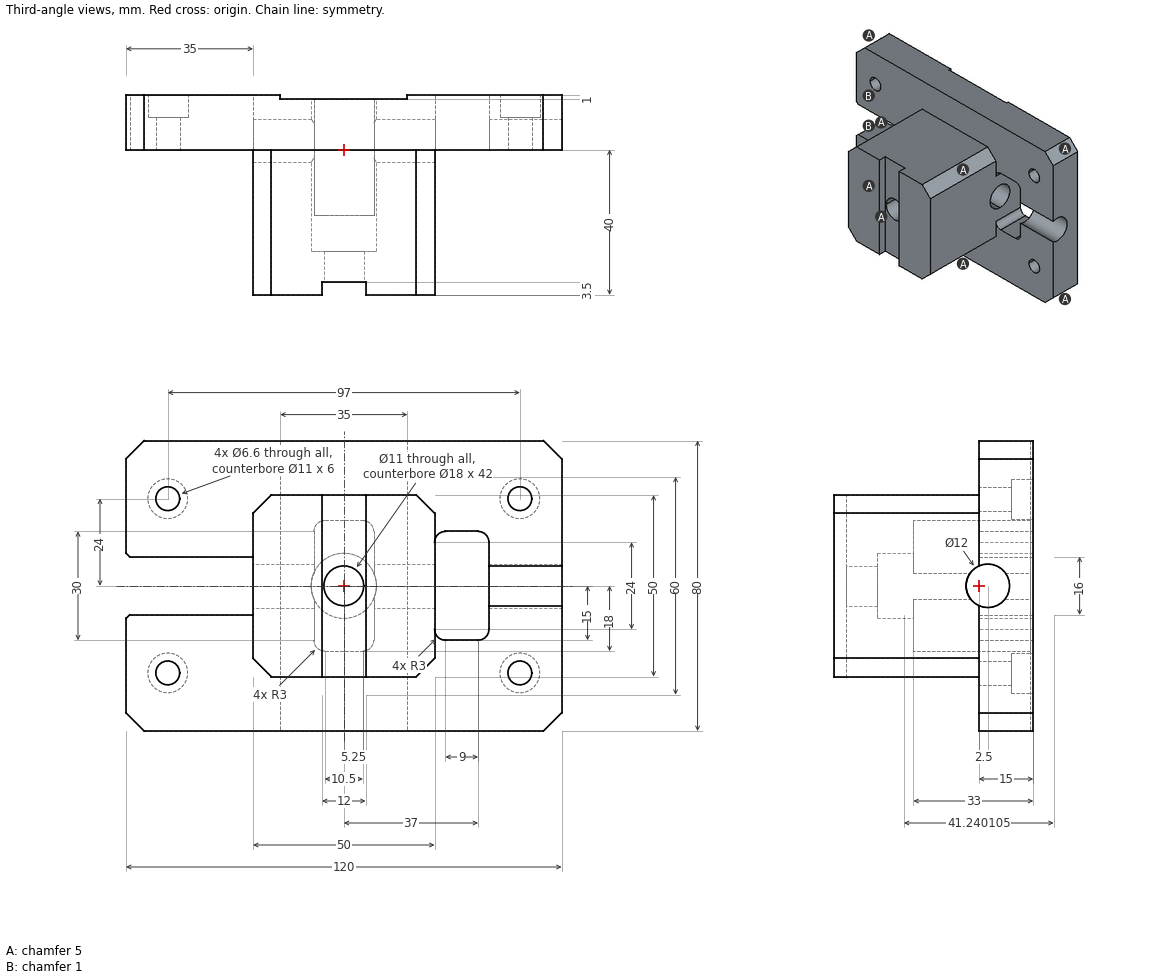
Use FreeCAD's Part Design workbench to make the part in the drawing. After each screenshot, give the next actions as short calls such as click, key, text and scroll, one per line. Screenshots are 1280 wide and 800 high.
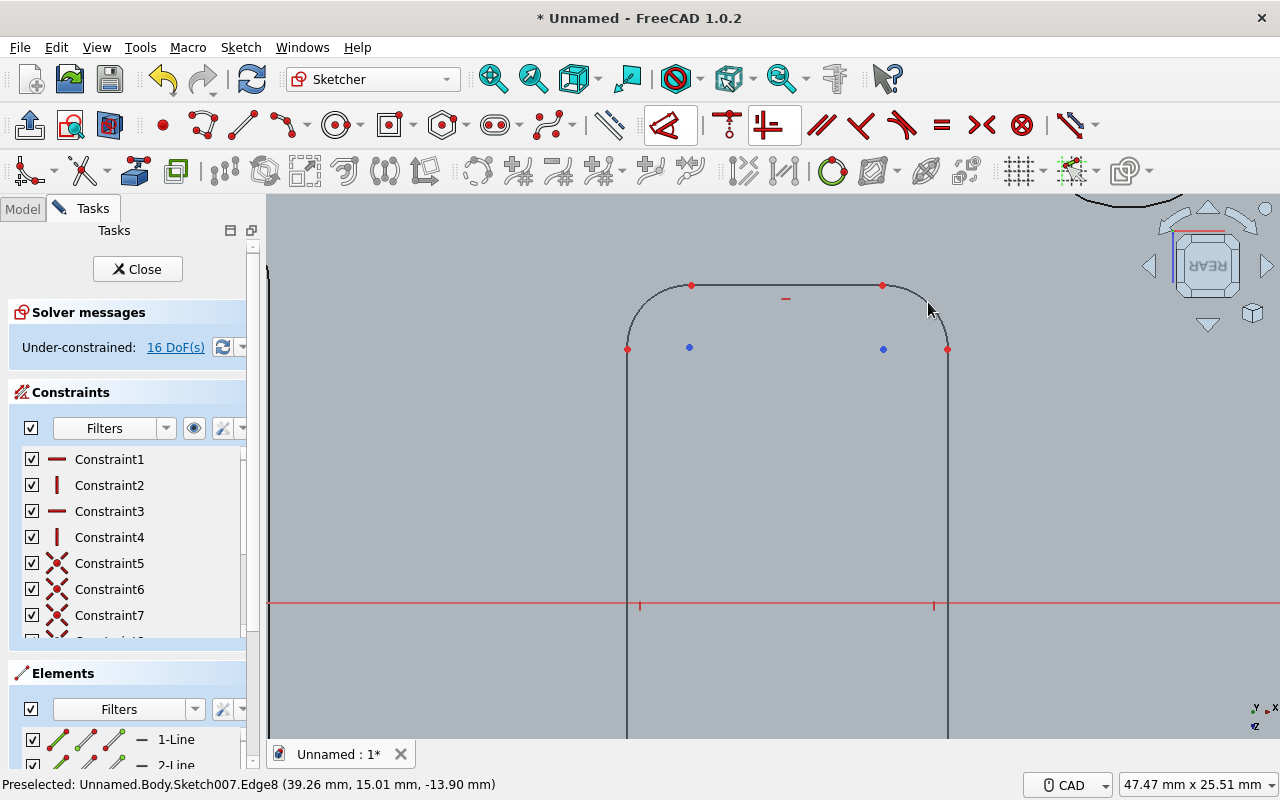
click(825, 285)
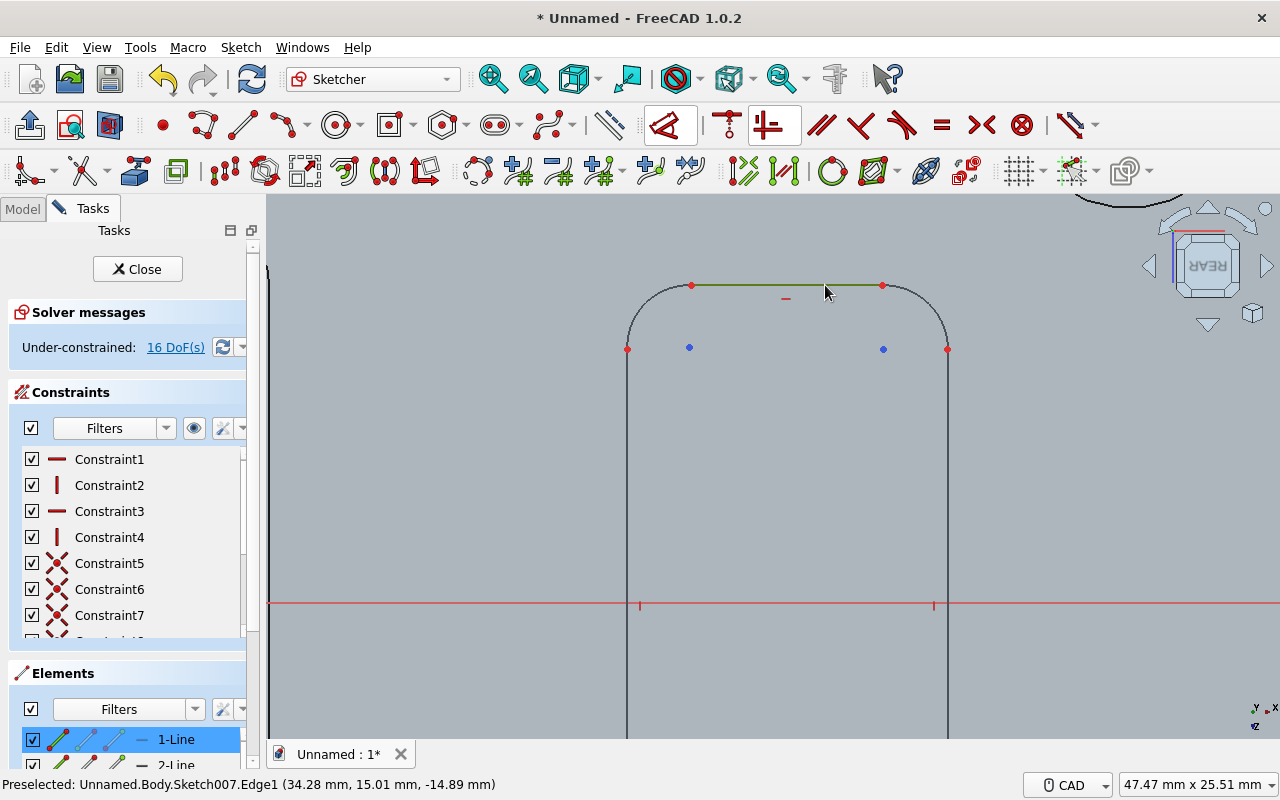
click(662, 292)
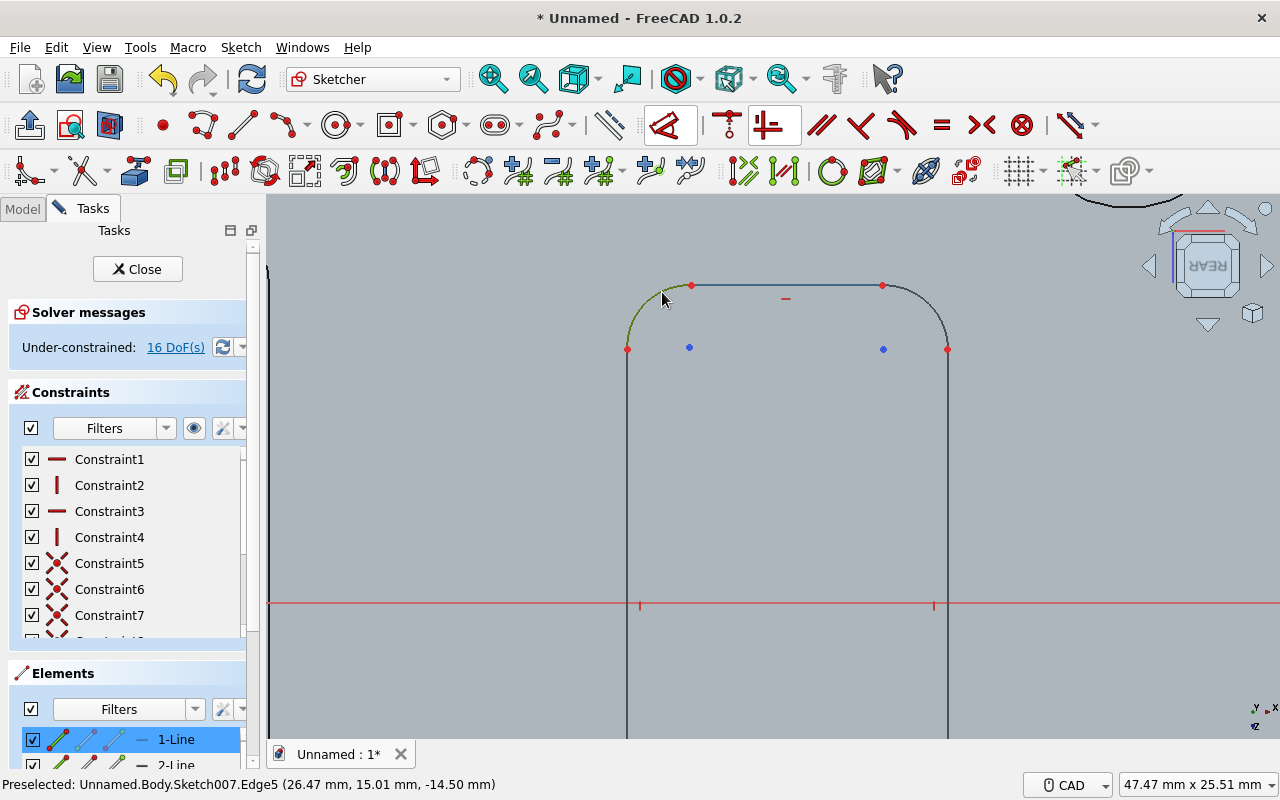
click(902, 126)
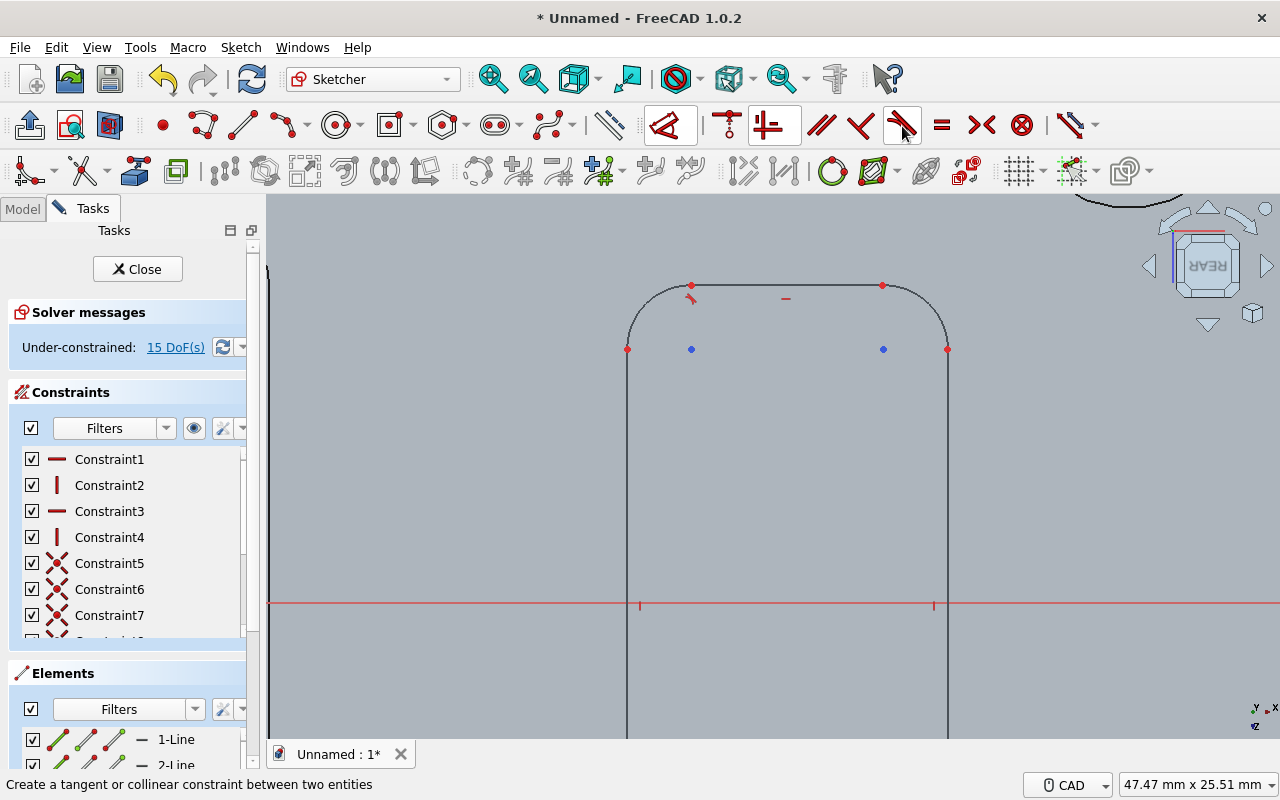
click(825, 285)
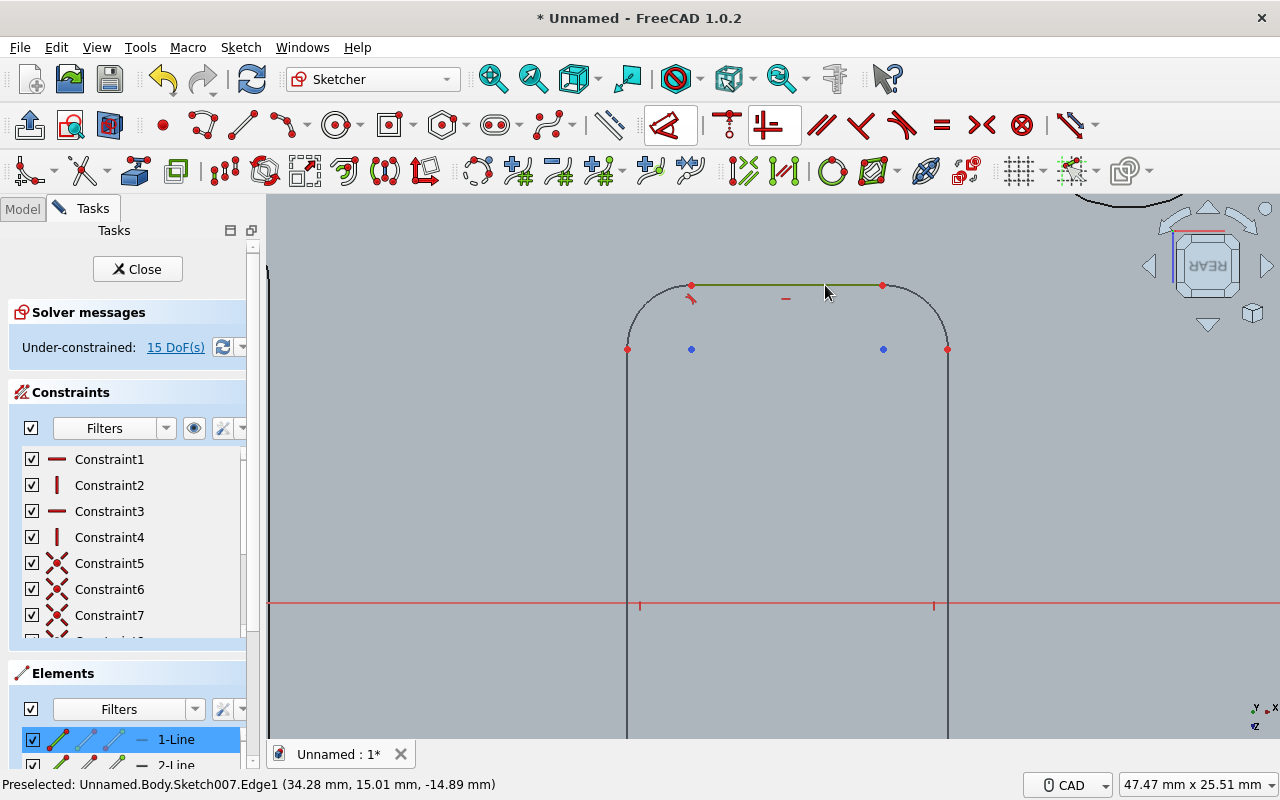
click(941, 320)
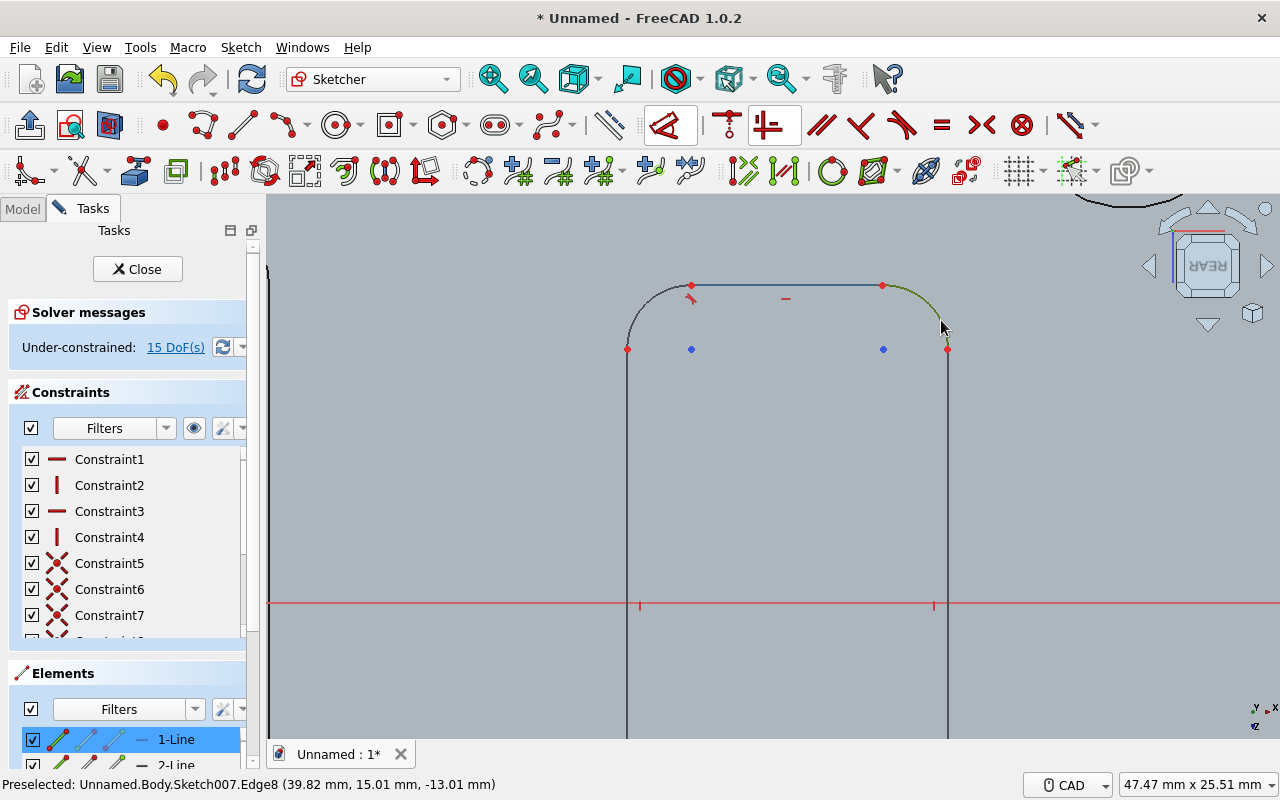
key(t)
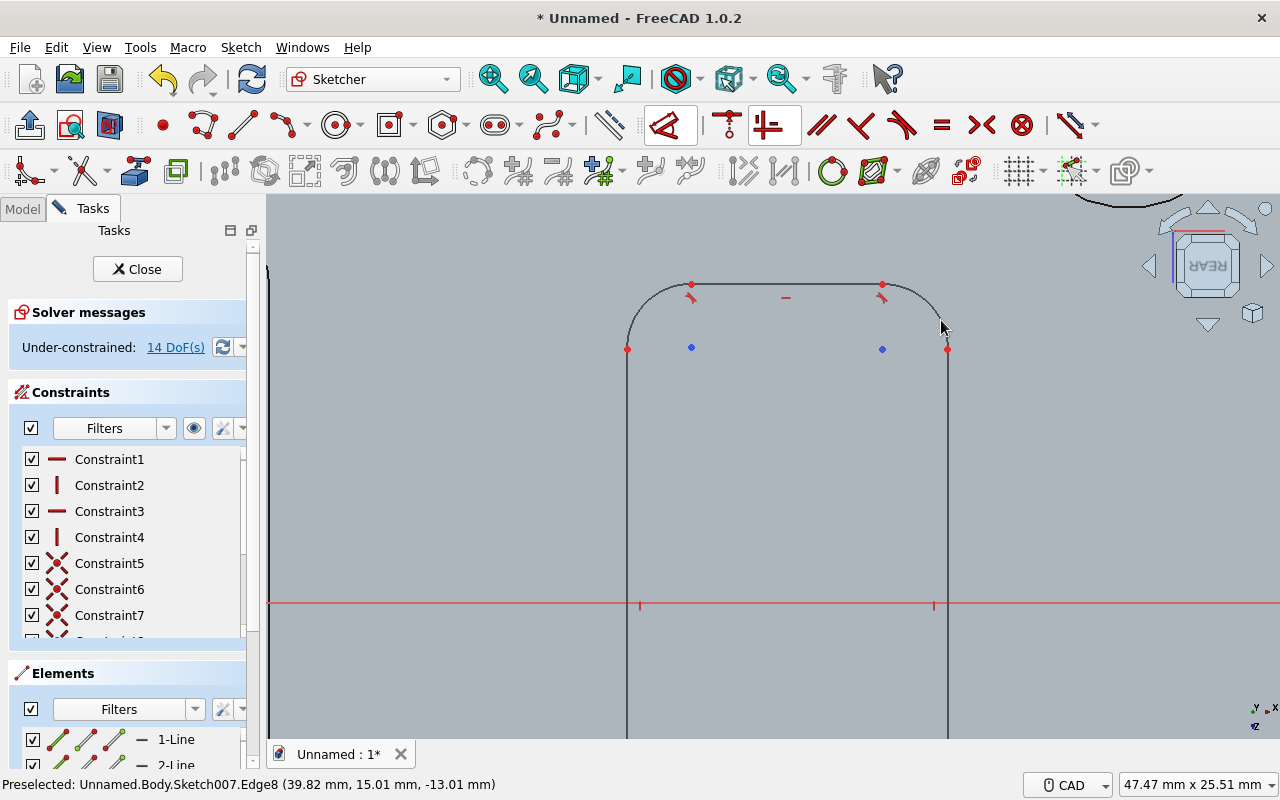
click(627, 503)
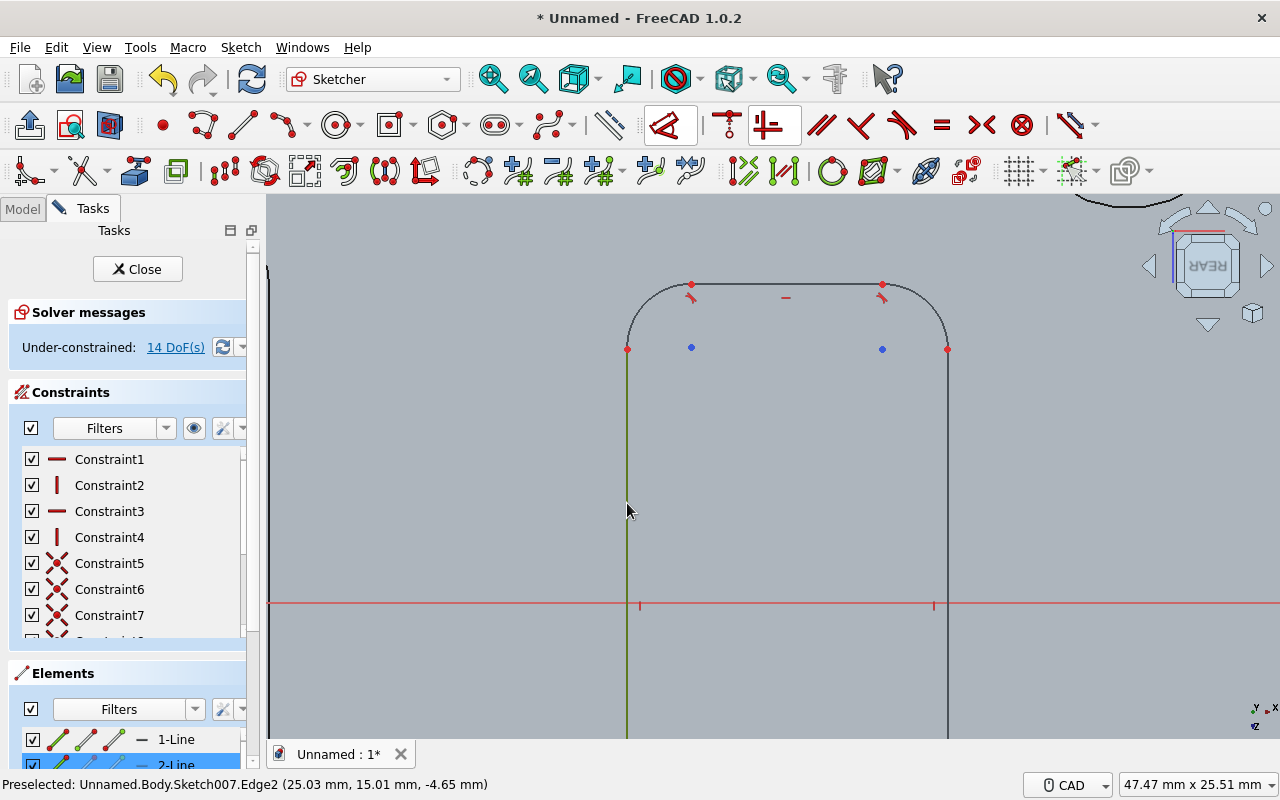
click(662, 291)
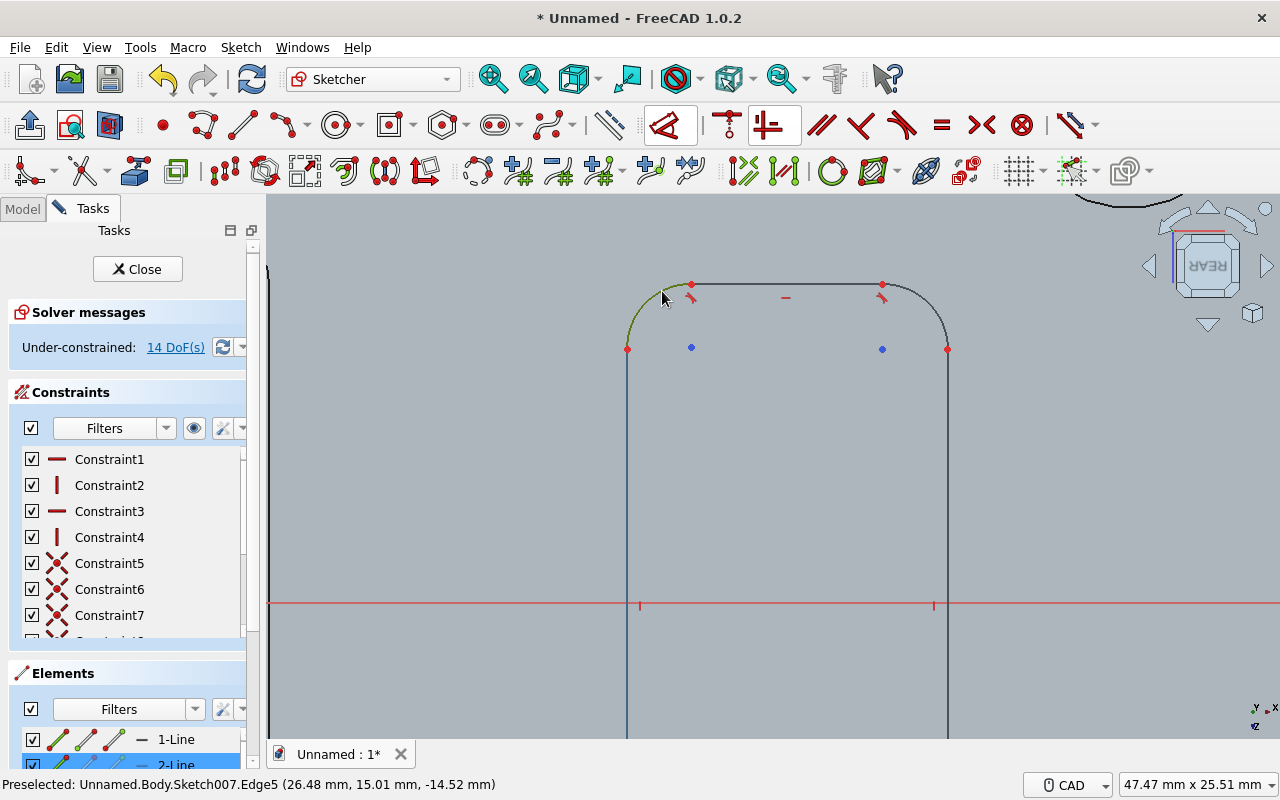
click(902, 126)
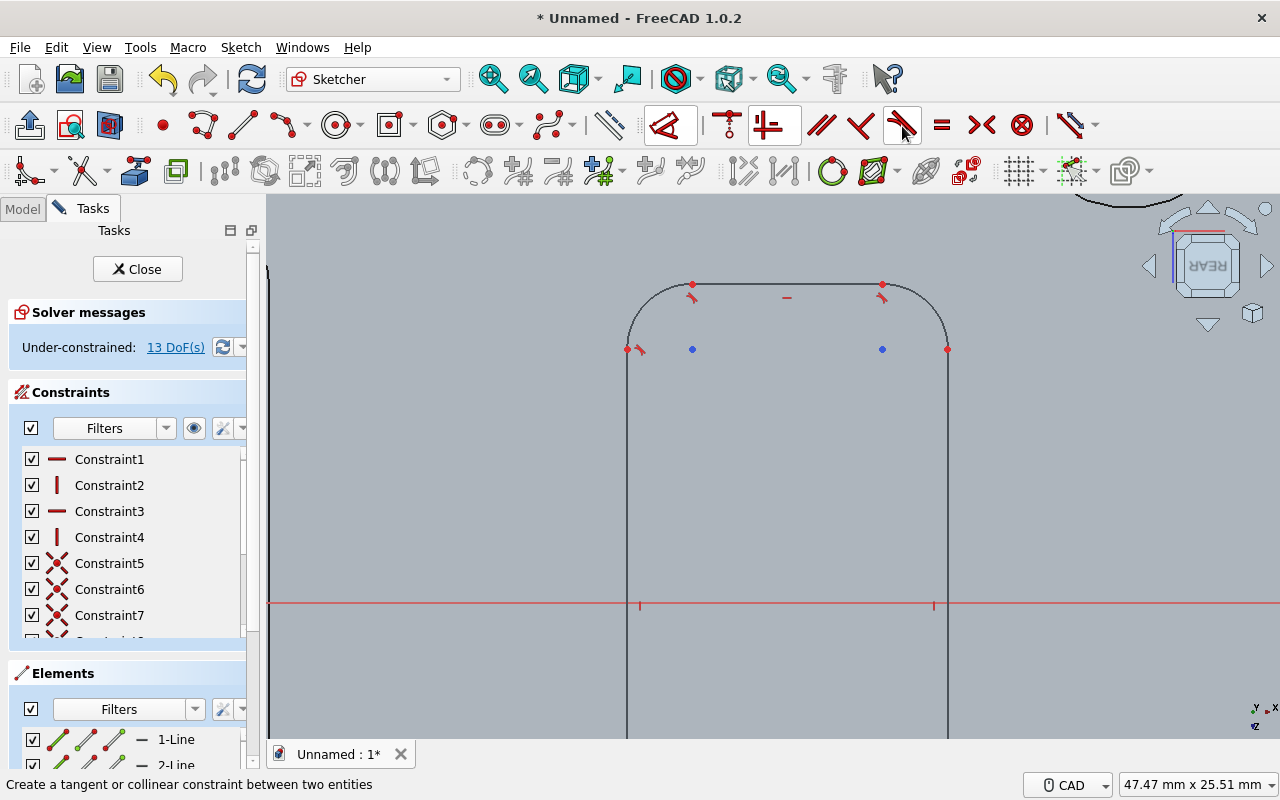
click(627, 503)